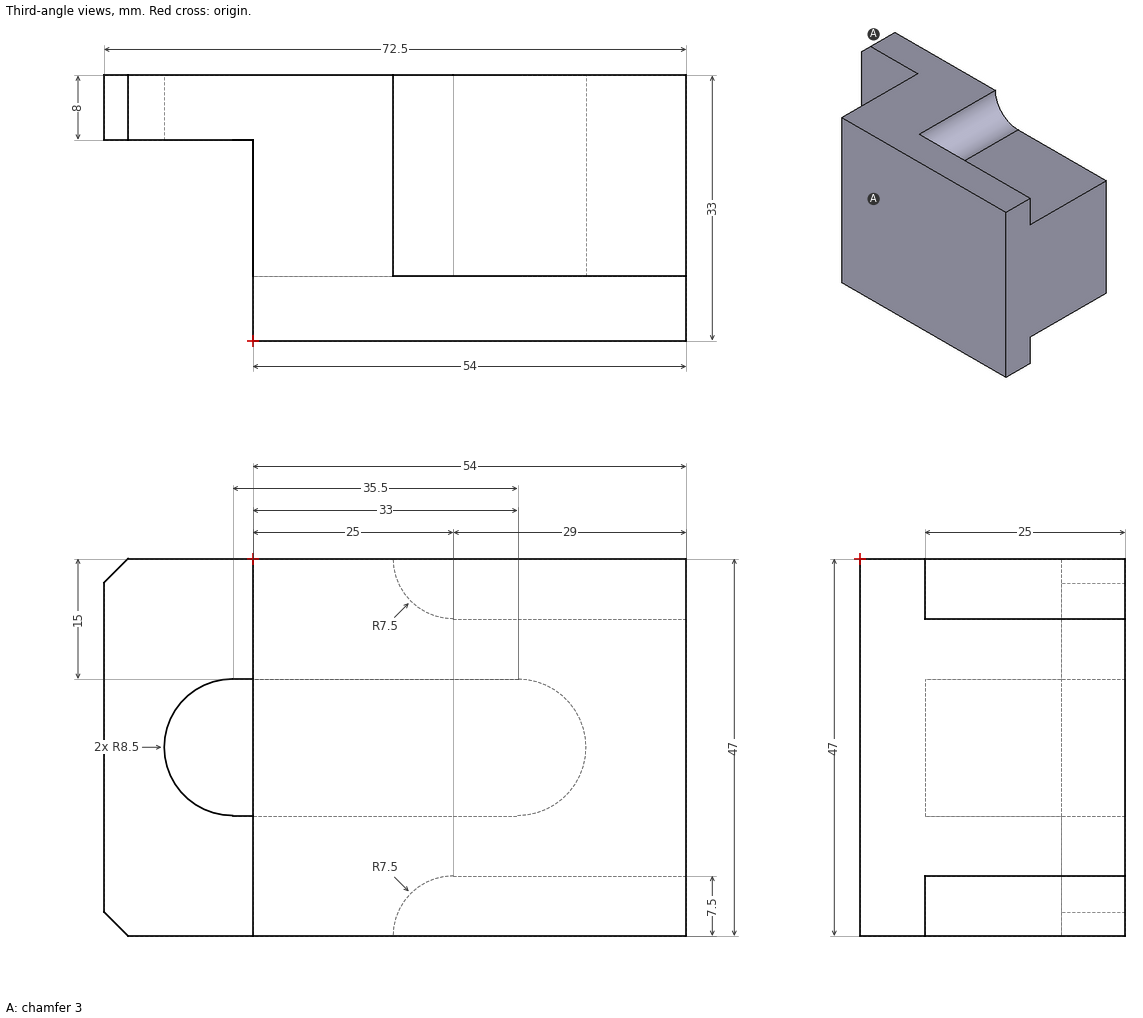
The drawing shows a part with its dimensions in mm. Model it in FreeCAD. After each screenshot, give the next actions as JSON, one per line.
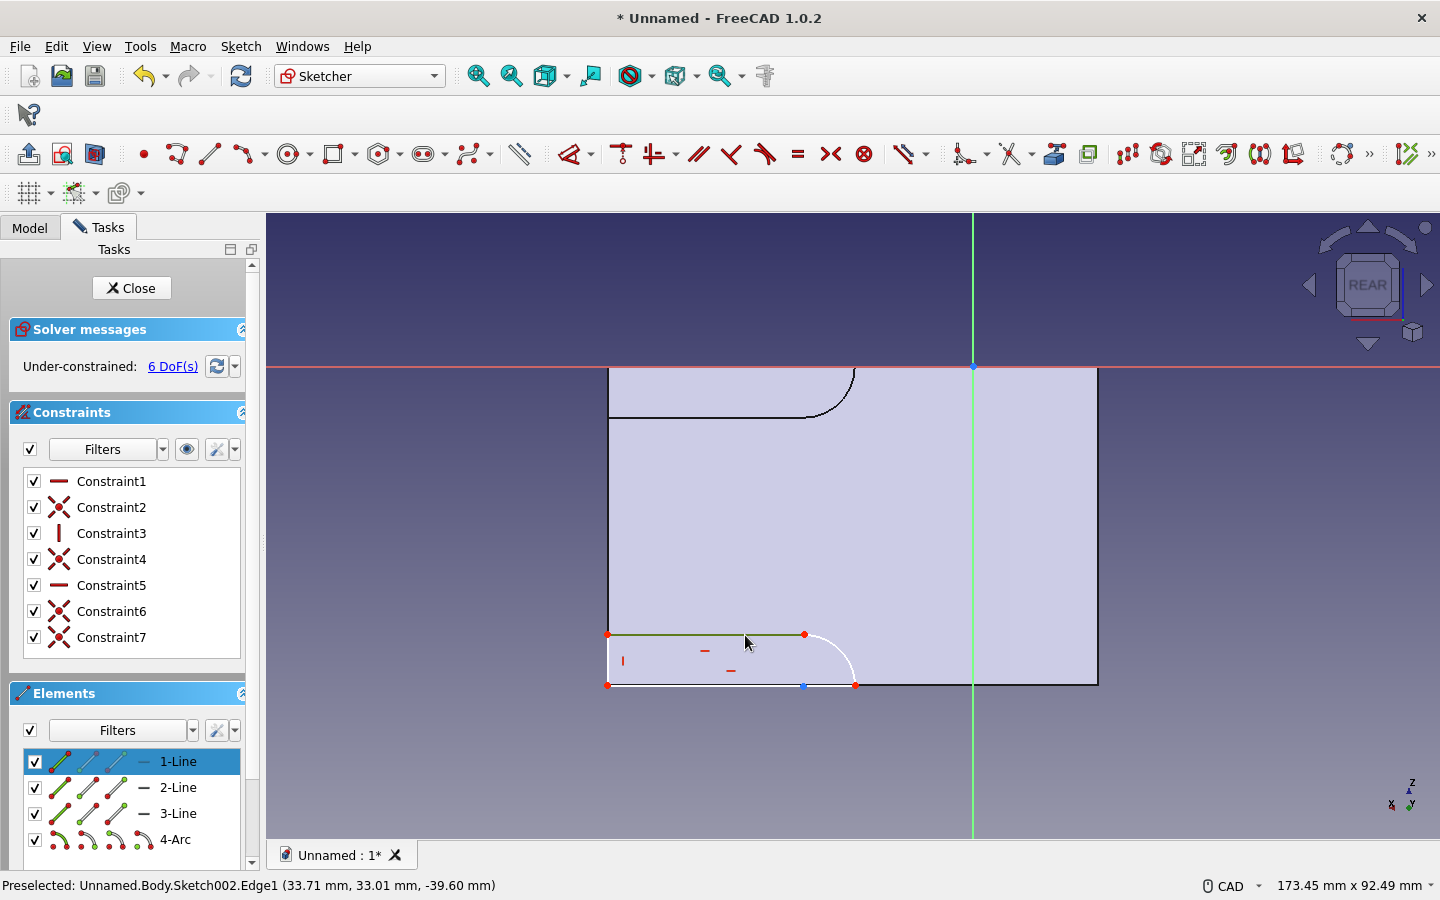
{"action": "left_click", "coordinate": [849, 663]}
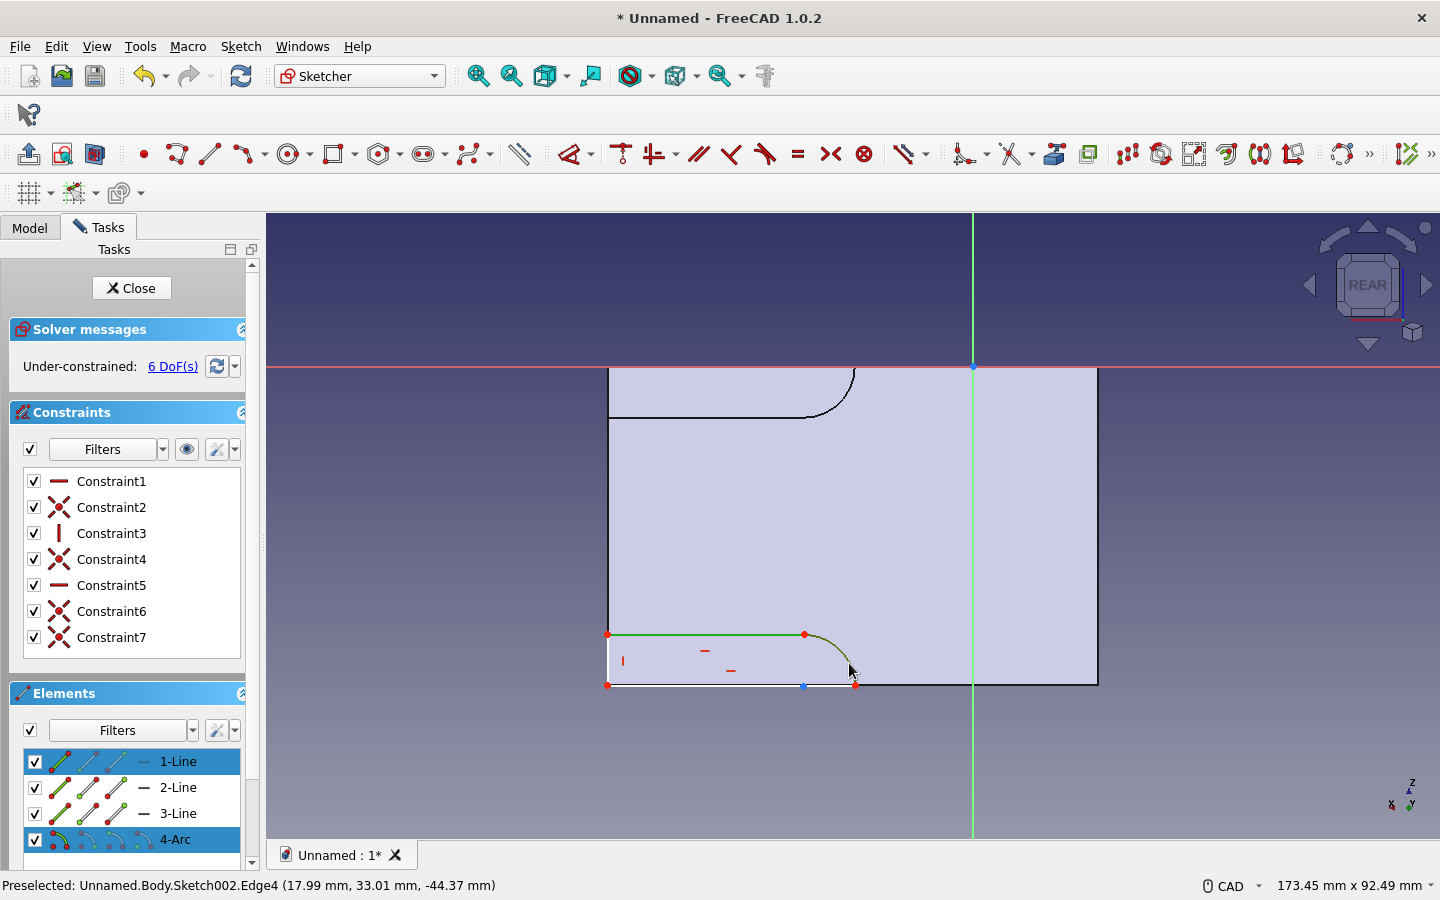
{"action": "key", "text": "t"}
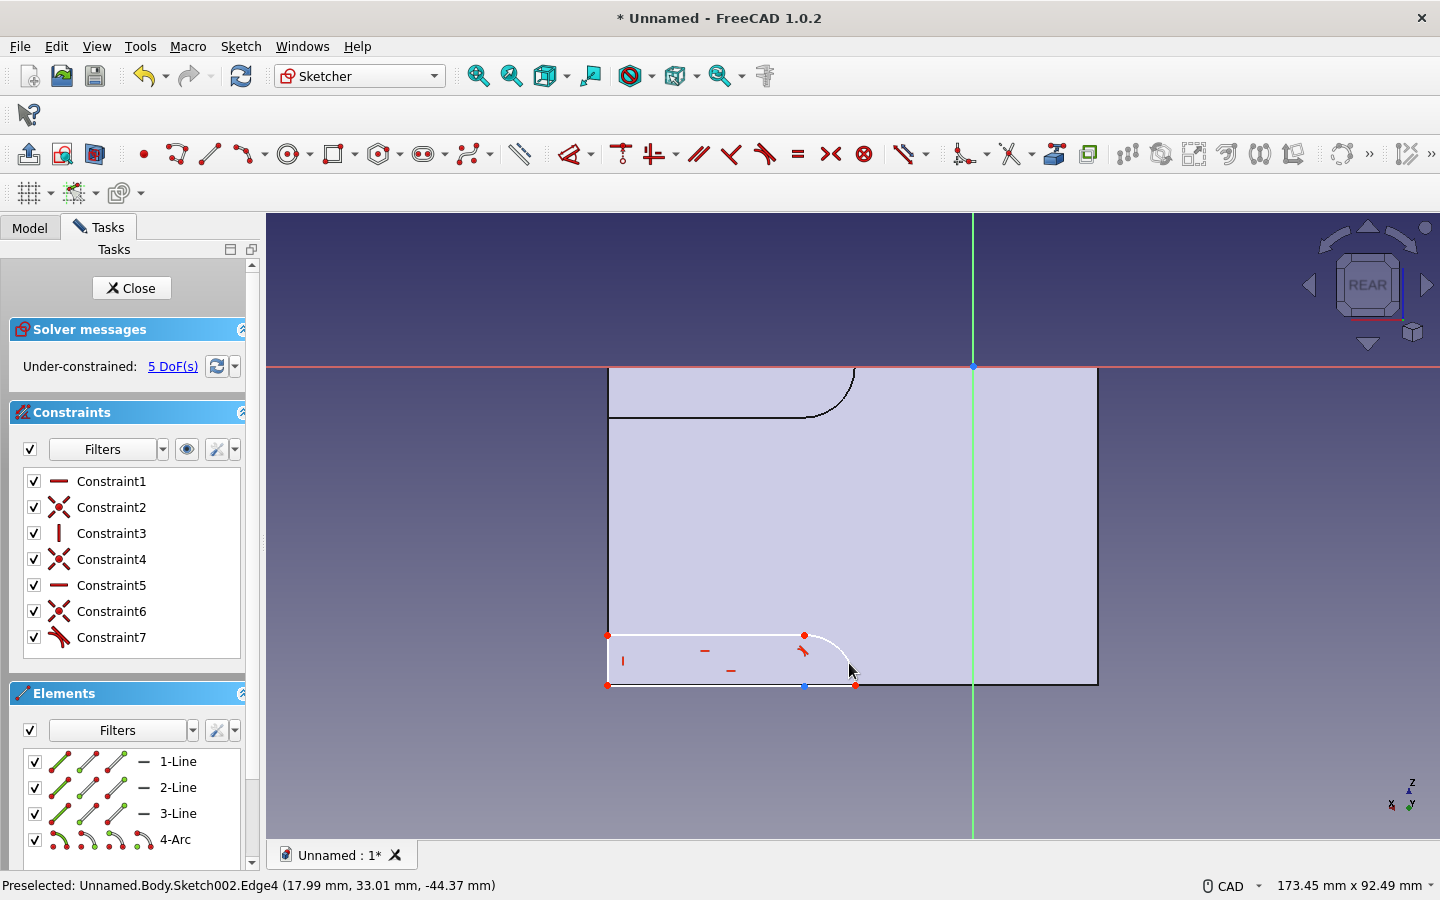
{"action": "key", "text": "d"}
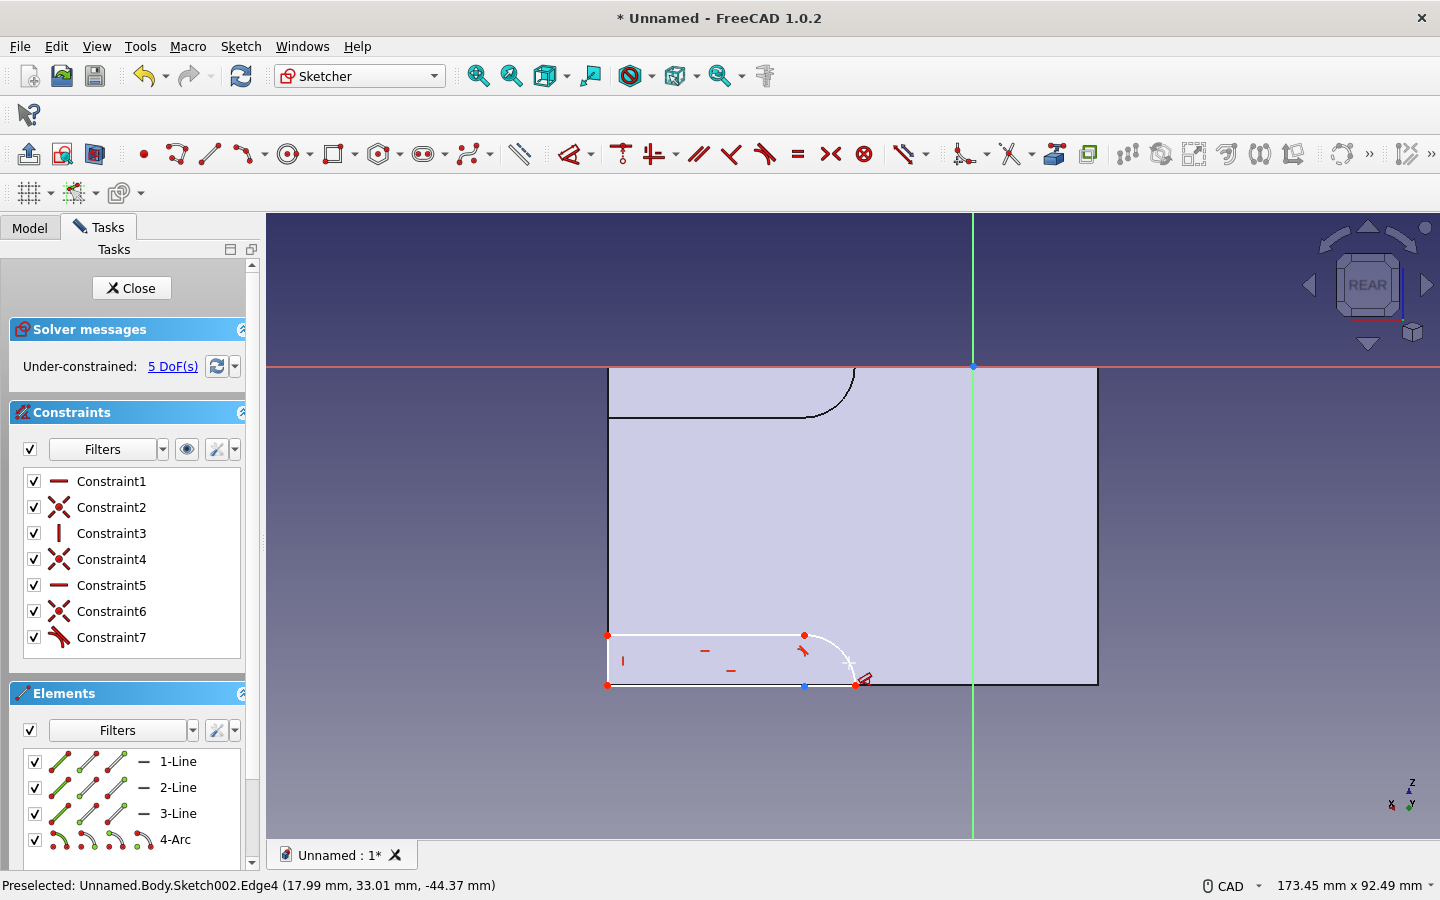
{"action": "left_click", "coordinate": [850, 663]}
{"action": "left_click", "coordinate": [879, 649]}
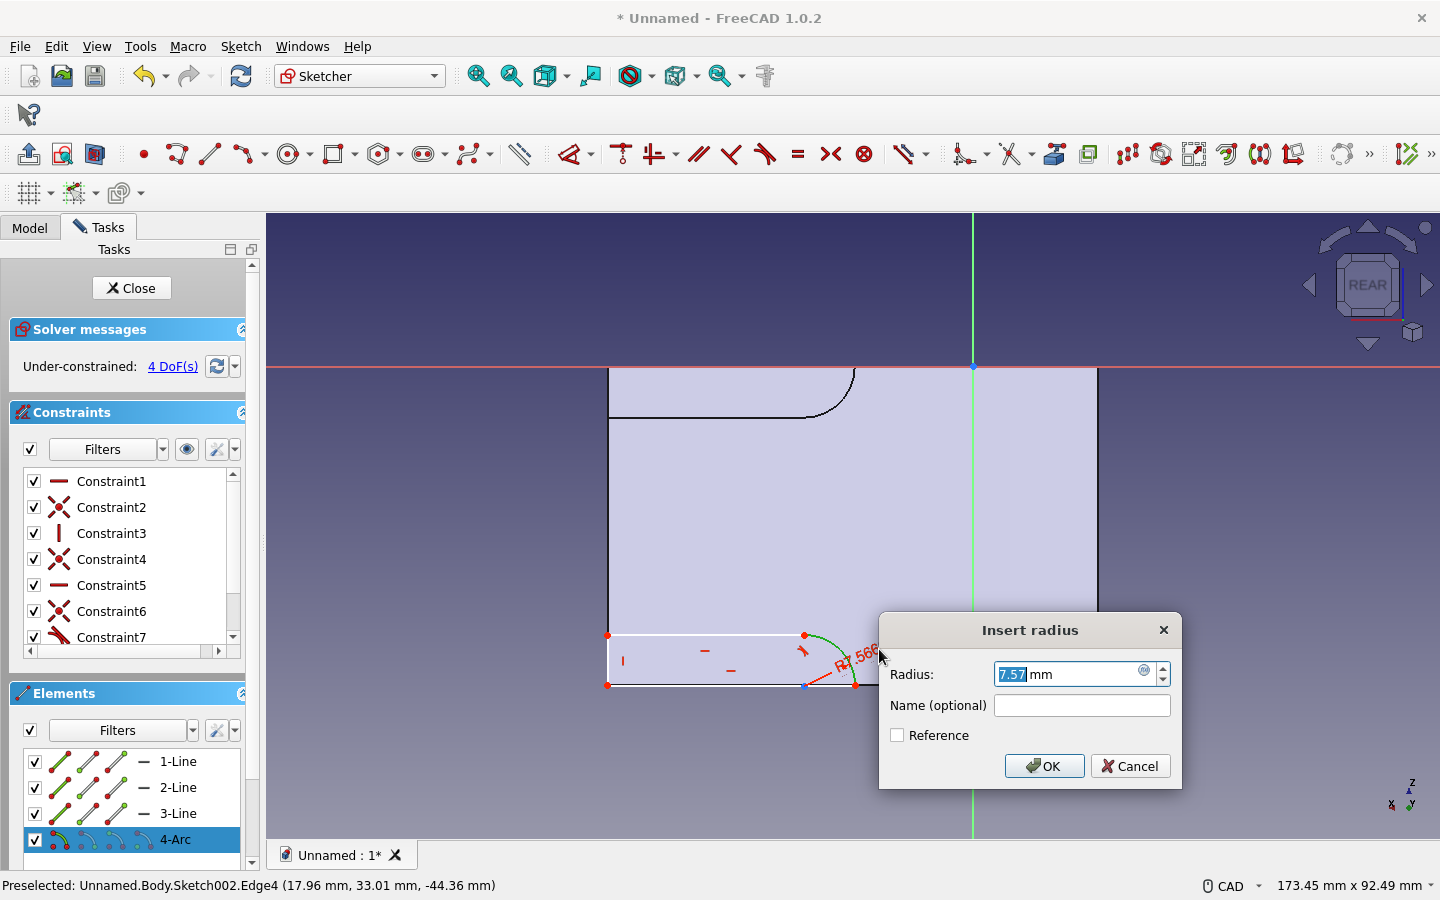
{"action": "type", "text": "7.5"}
{"action": "key", "text": "Return"}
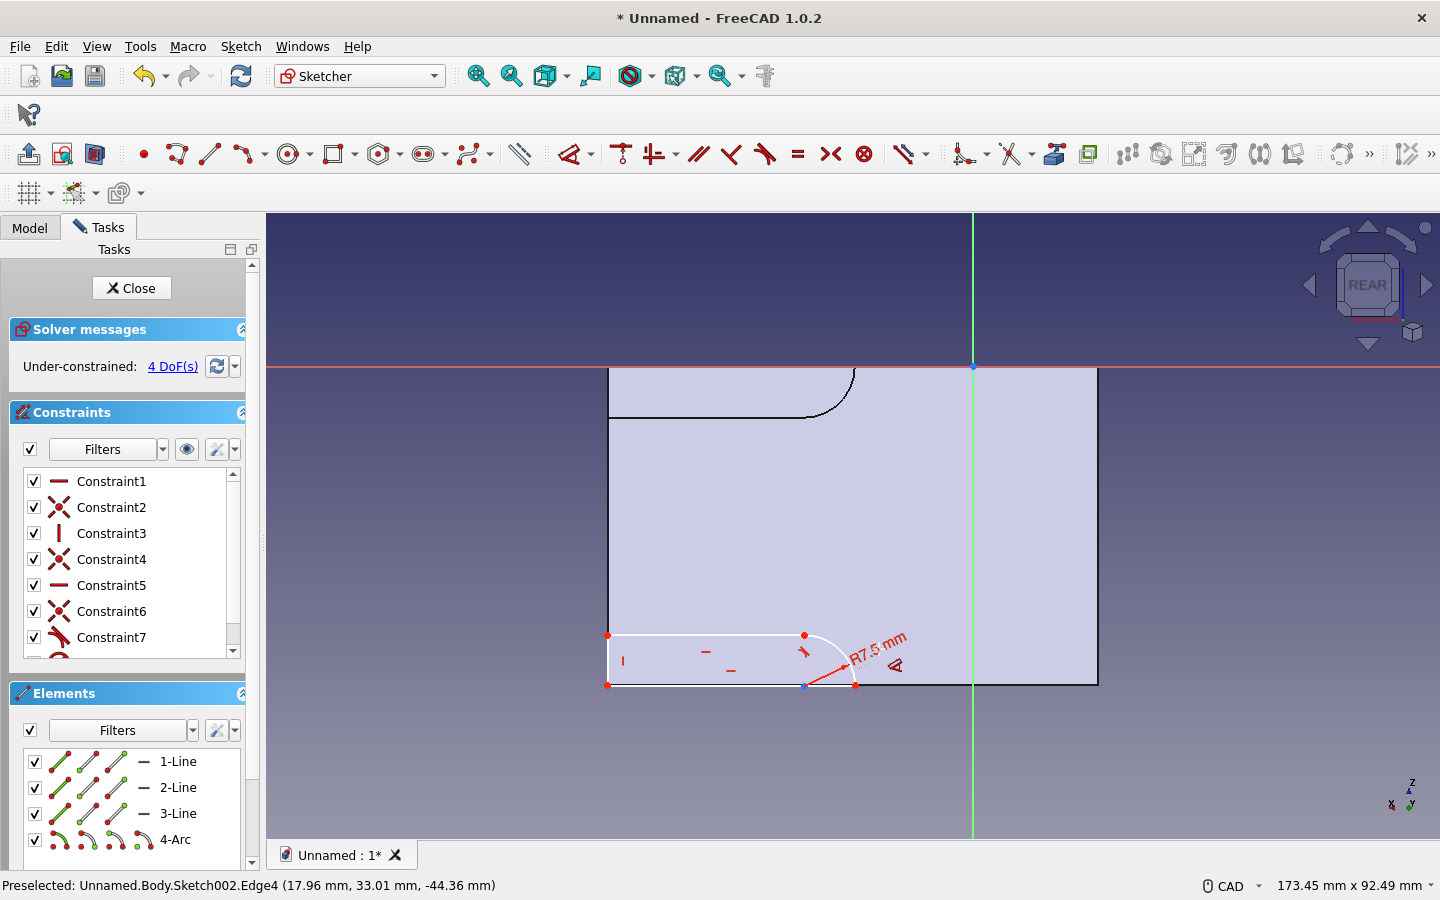
{"action": "left_click", "coordinate": [746, 635]}
{"action": "left_click", "coordinate": [706, 669]}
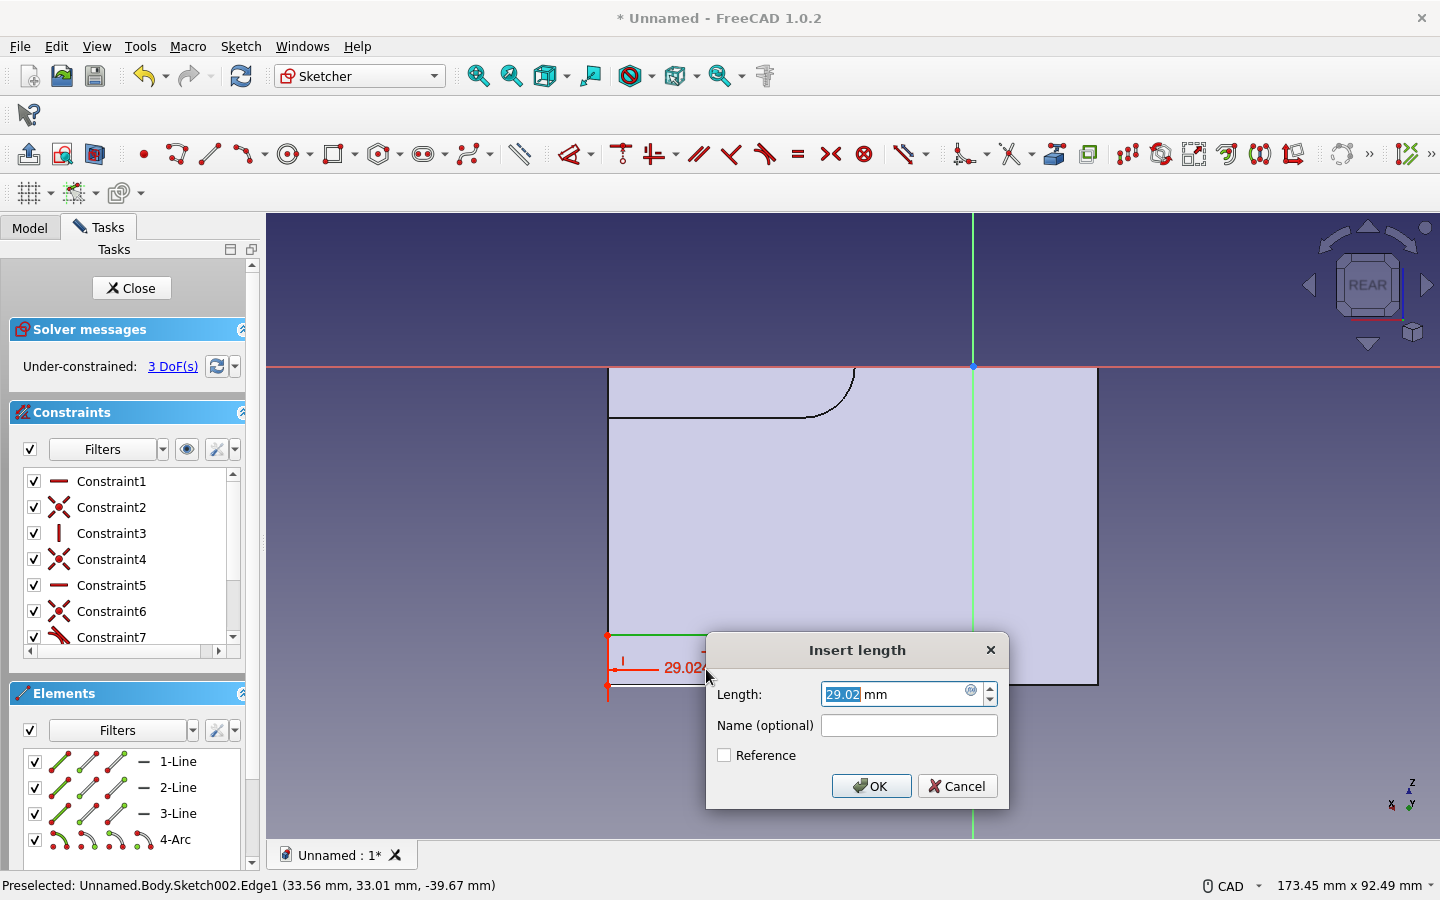
{"action": "type", "text": "29"}
{"action": "key", "text": "Return"}